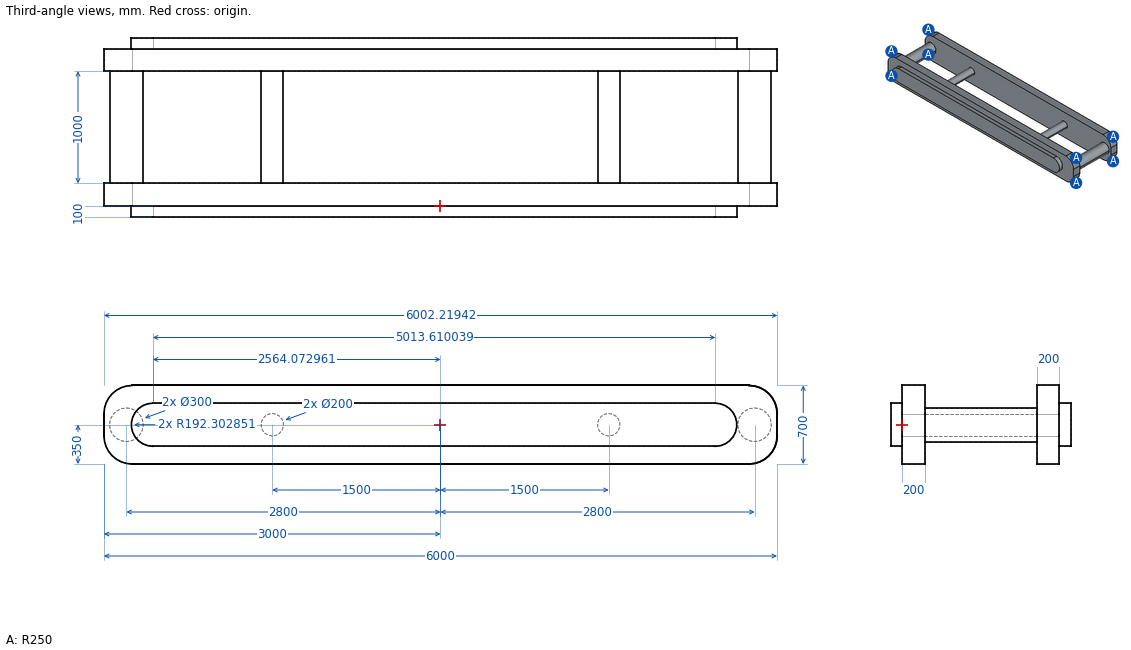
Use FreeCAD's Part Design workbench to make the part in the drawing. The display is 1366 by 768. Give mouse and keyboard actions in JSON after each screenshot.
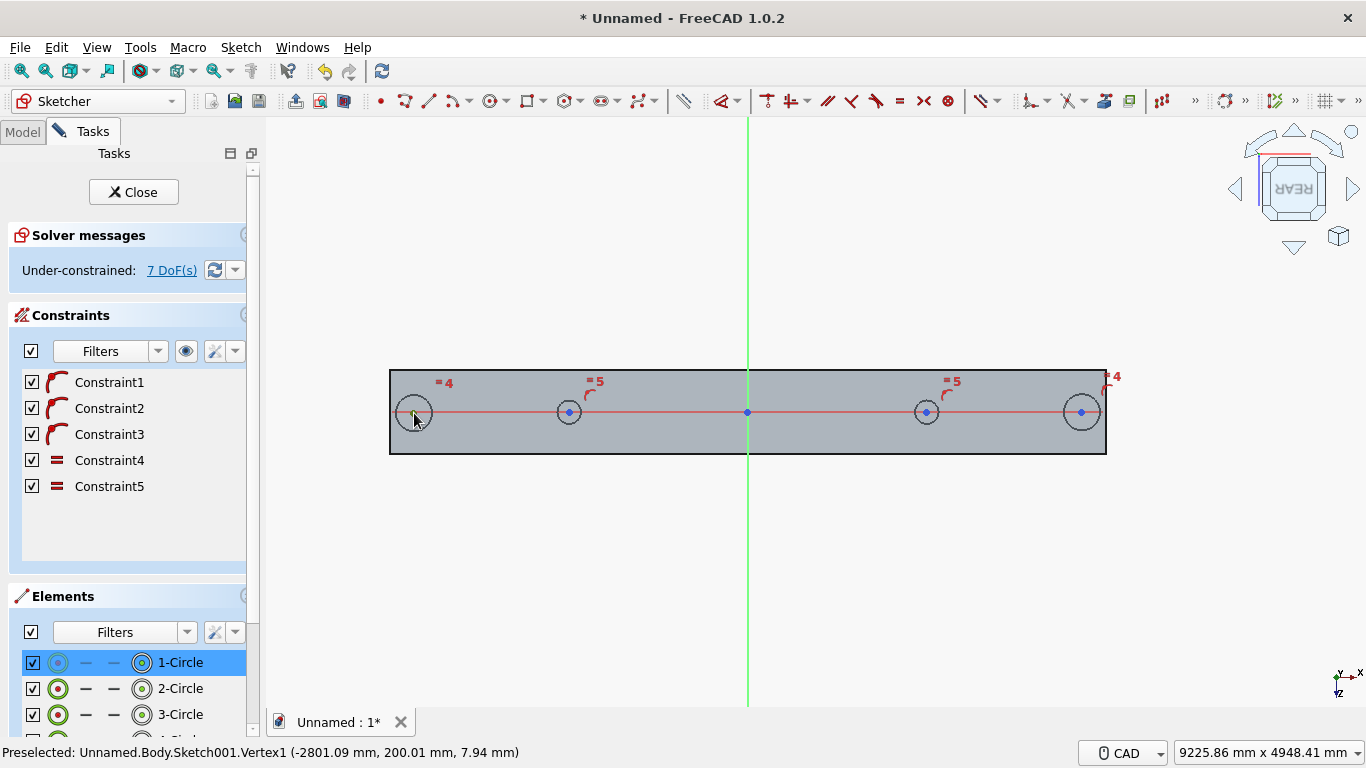
{"action": "left_click", "coordinate": [488, 412]}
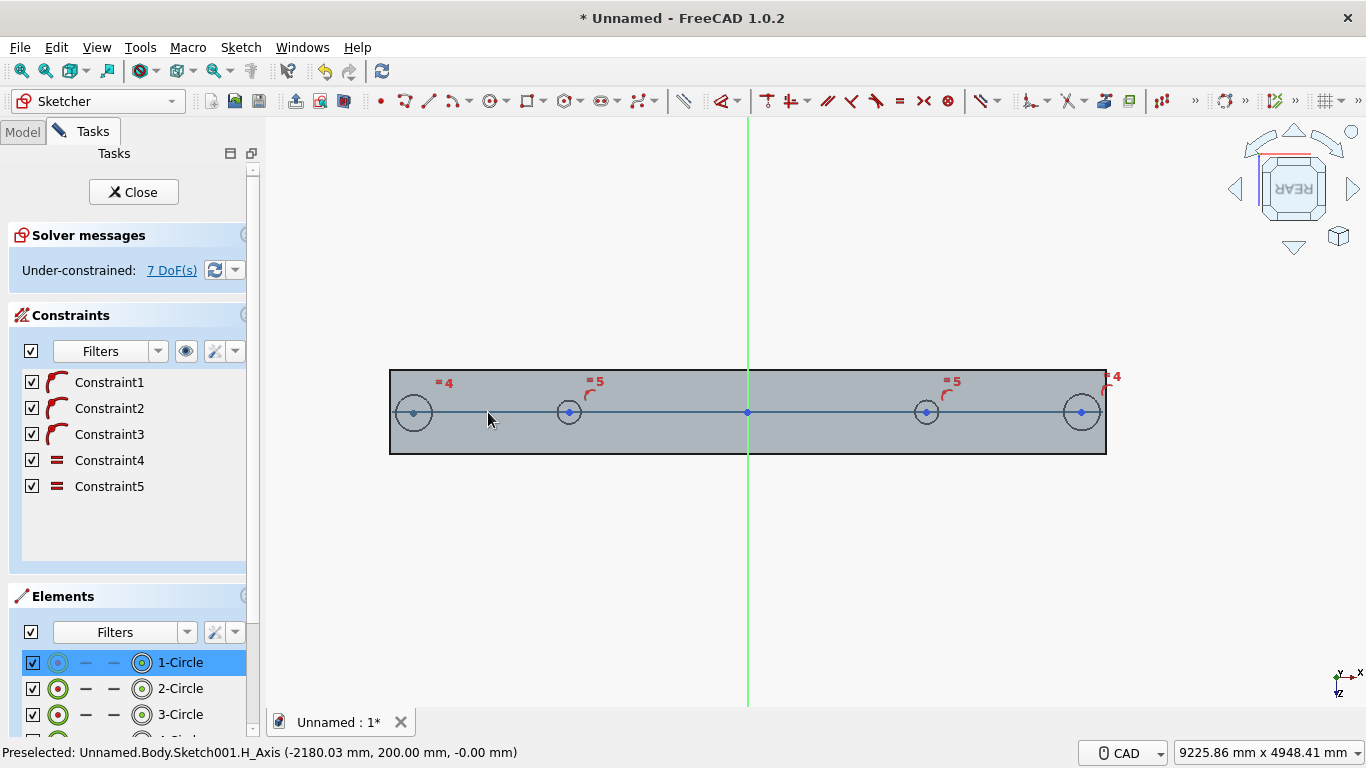
{"action": "left_click", "coordinate": [768, 102]}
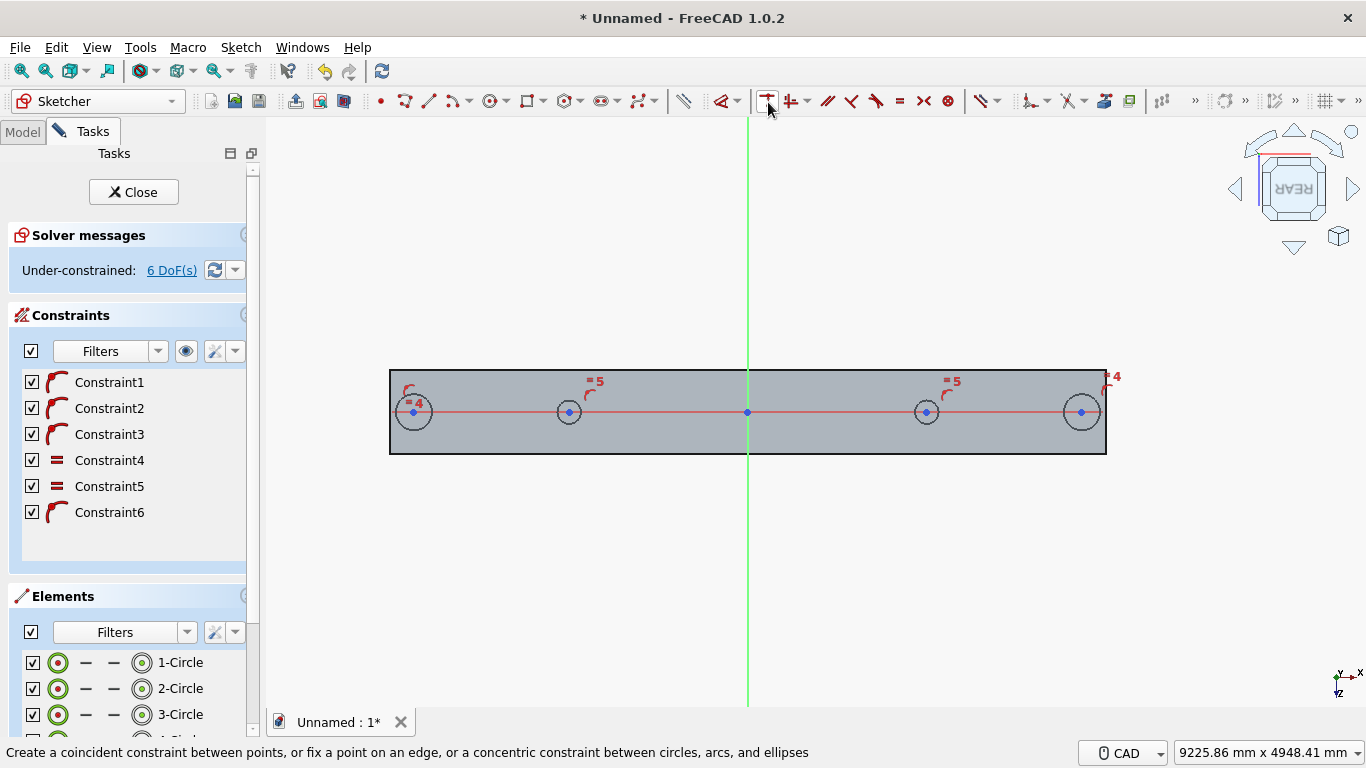
{"action": "left_click", "coordinate": [427, 399]}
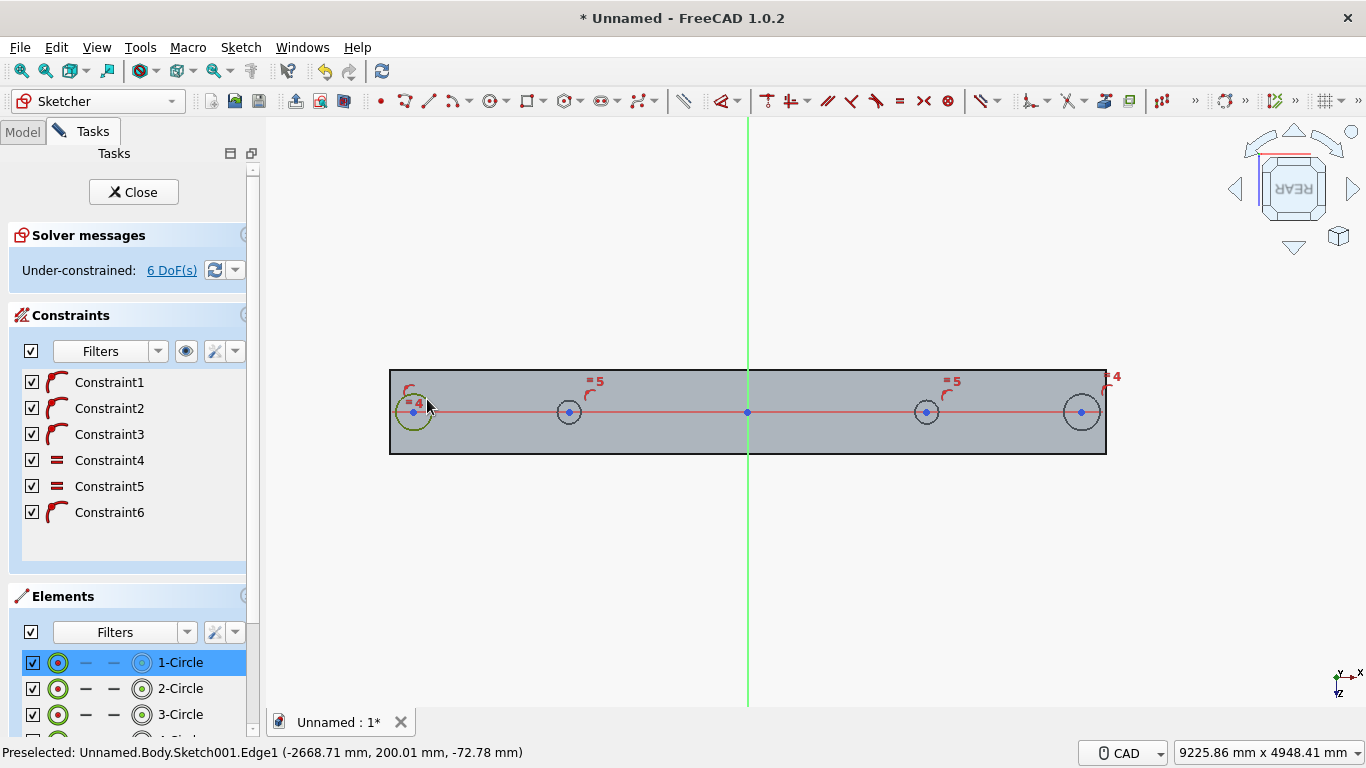
{"action": "key", "text": "k o"}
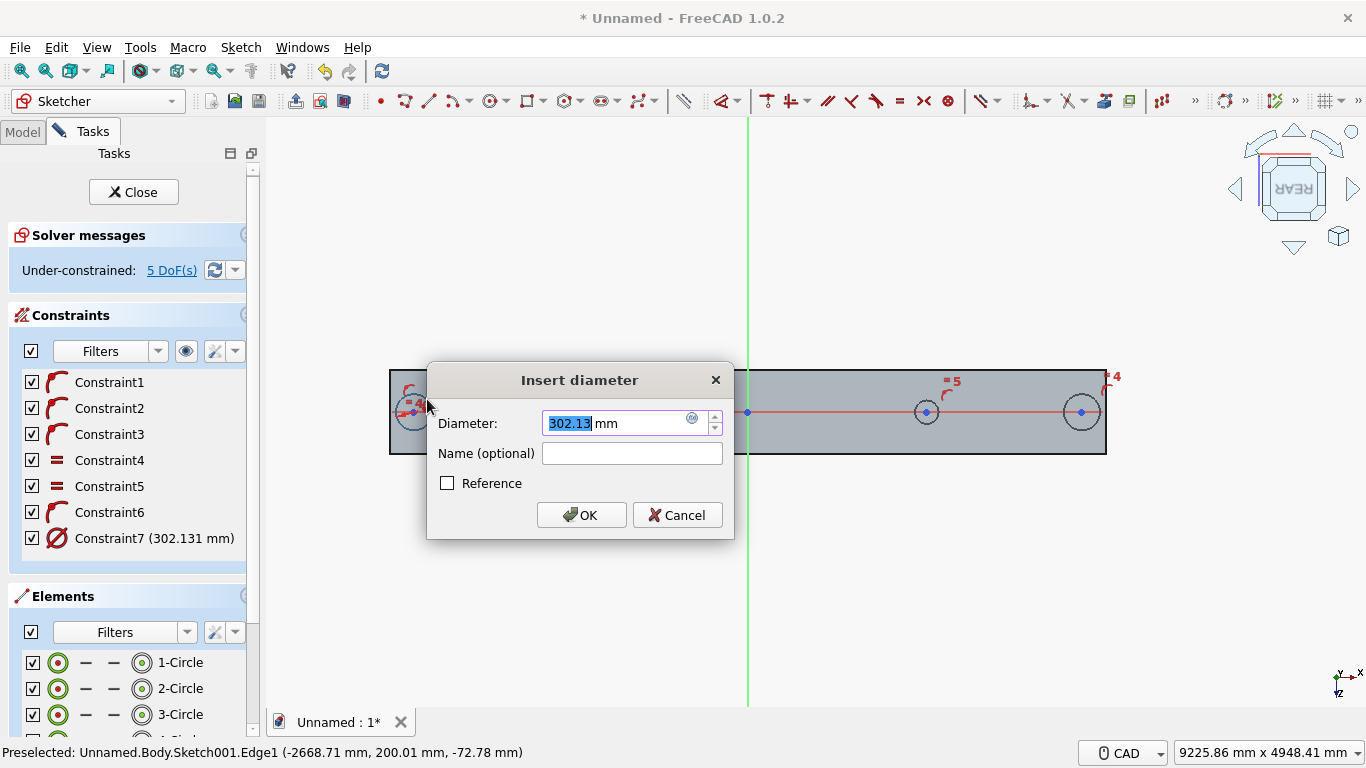
{"action": "type", "text": "300"}
{"action": "key", "text": "Return"}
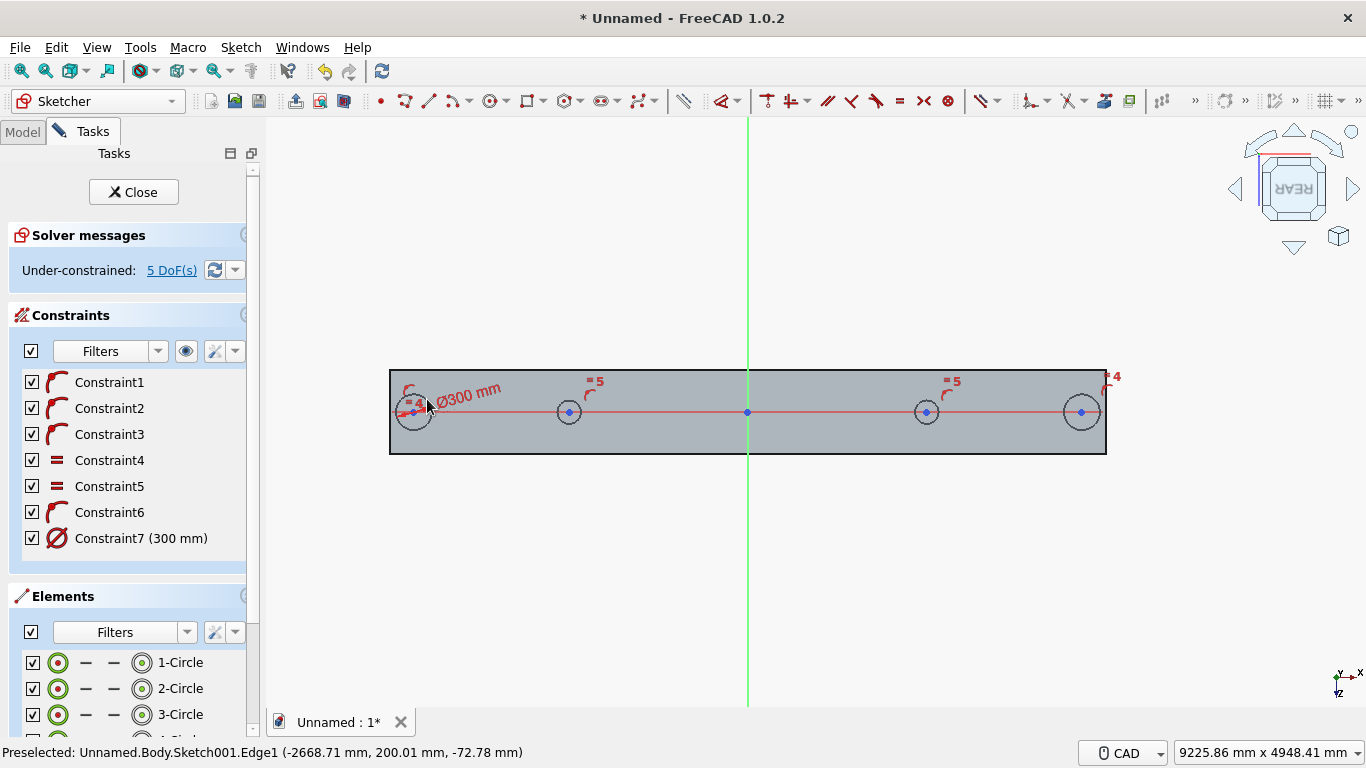
{"action": "scroll", "coordinate": [570, 401], "scroll_direction": "up", "scroll_amount": 3}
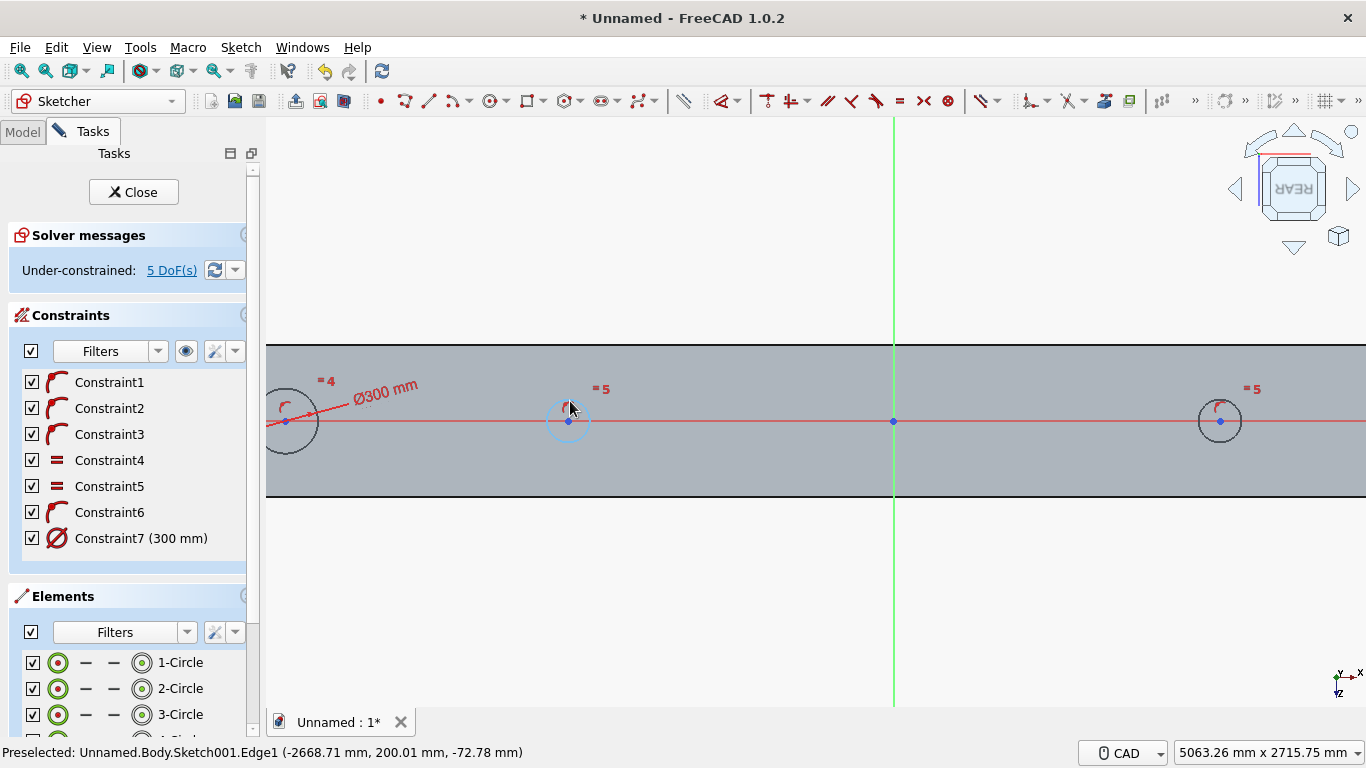
{"action": "left_click", "coordinate": [547, 420]}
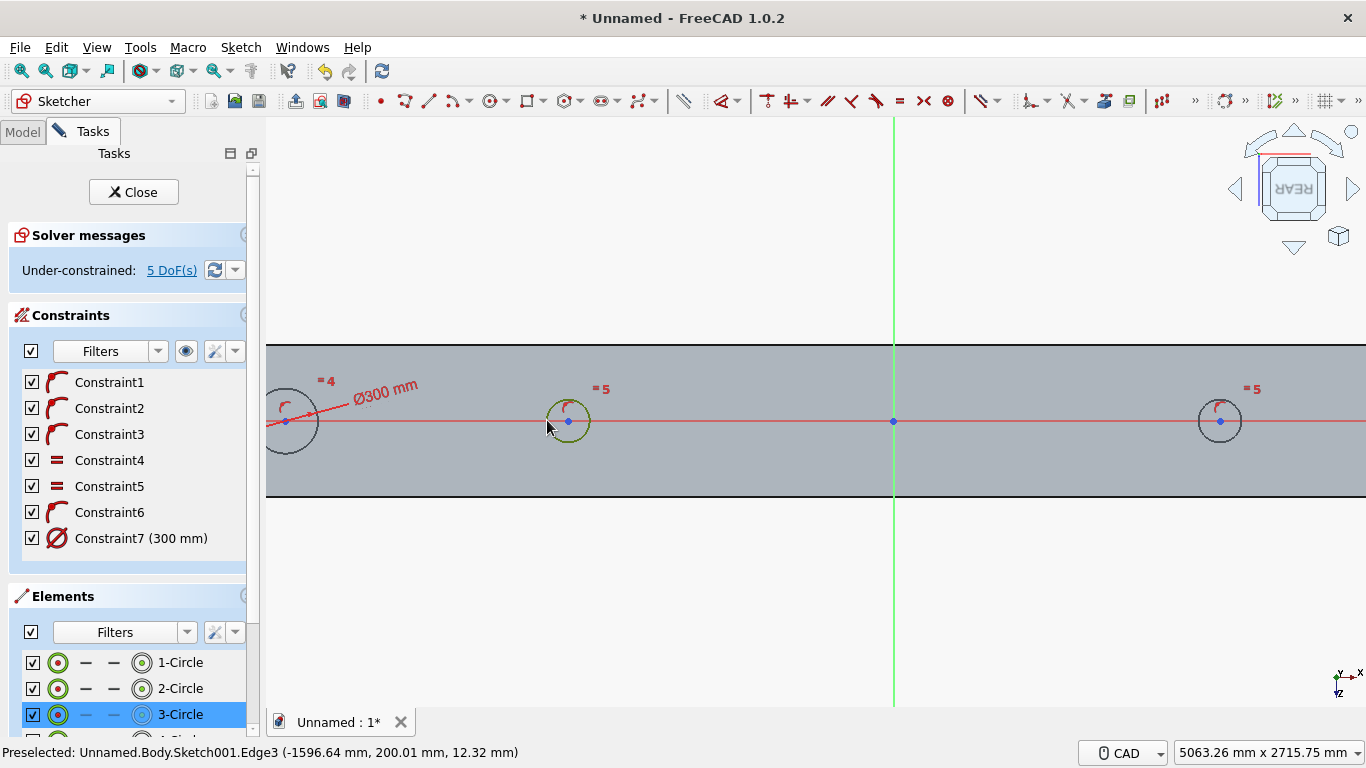
{"action": "key", "text": "k o"}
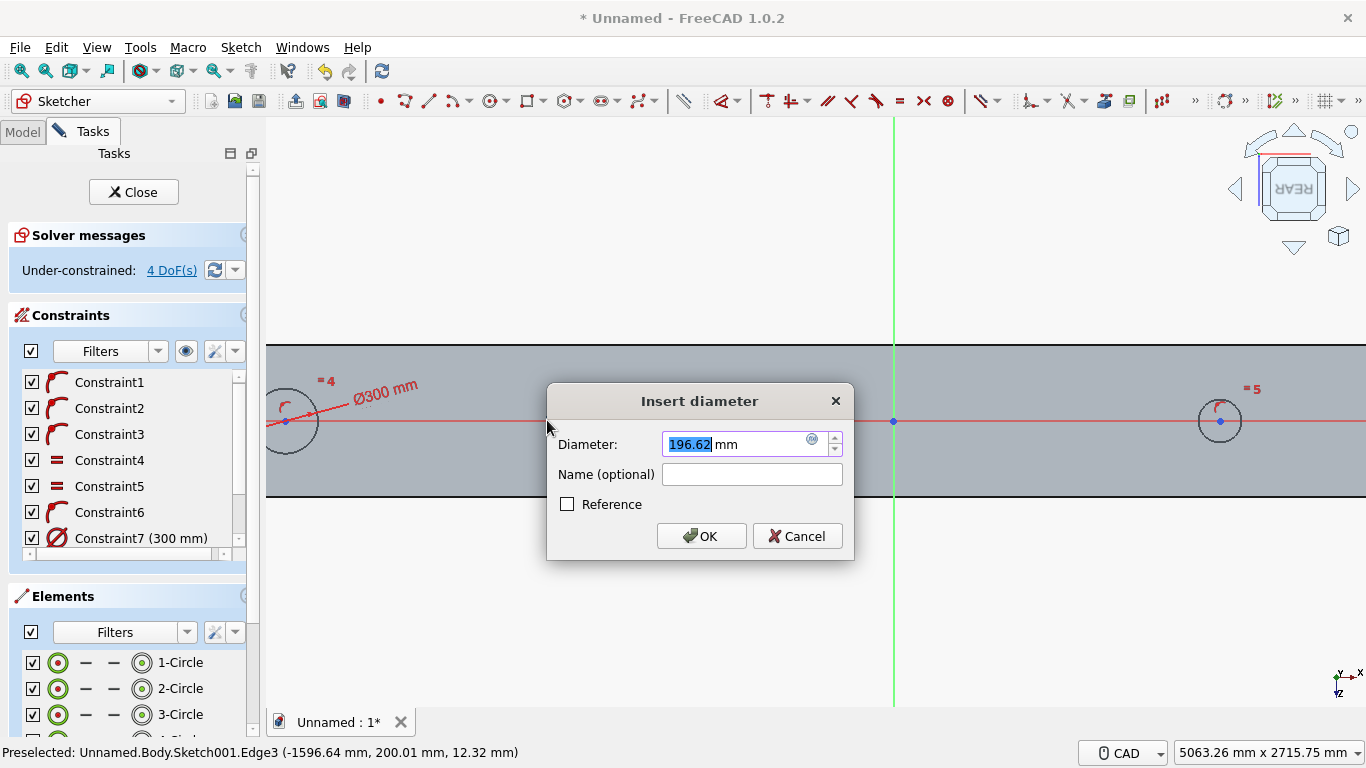
{"action": "type", "text": "200"}
{"action": "key", "text": "Return"}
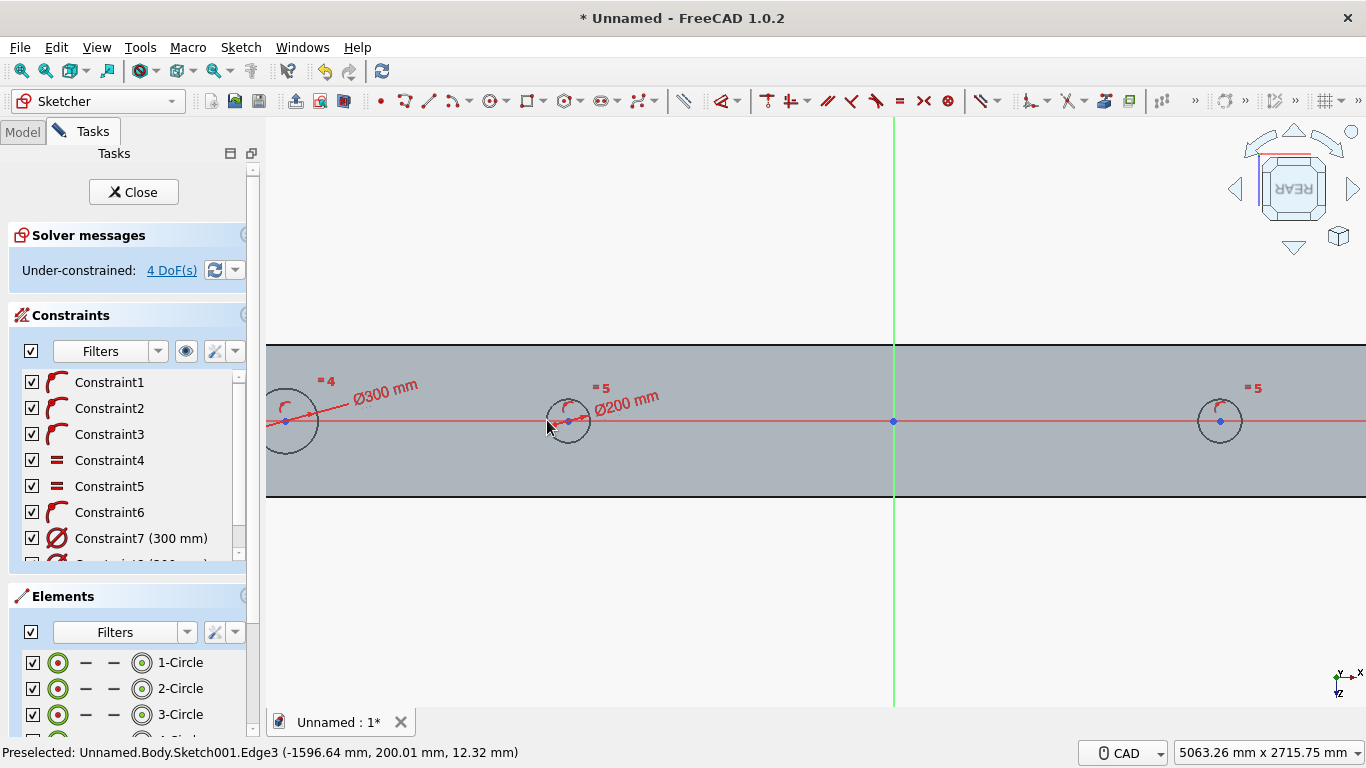
{"action": "scroll", "coordinate": [569, 401], "scroll_direction": "down", "scroll_amount": 3}